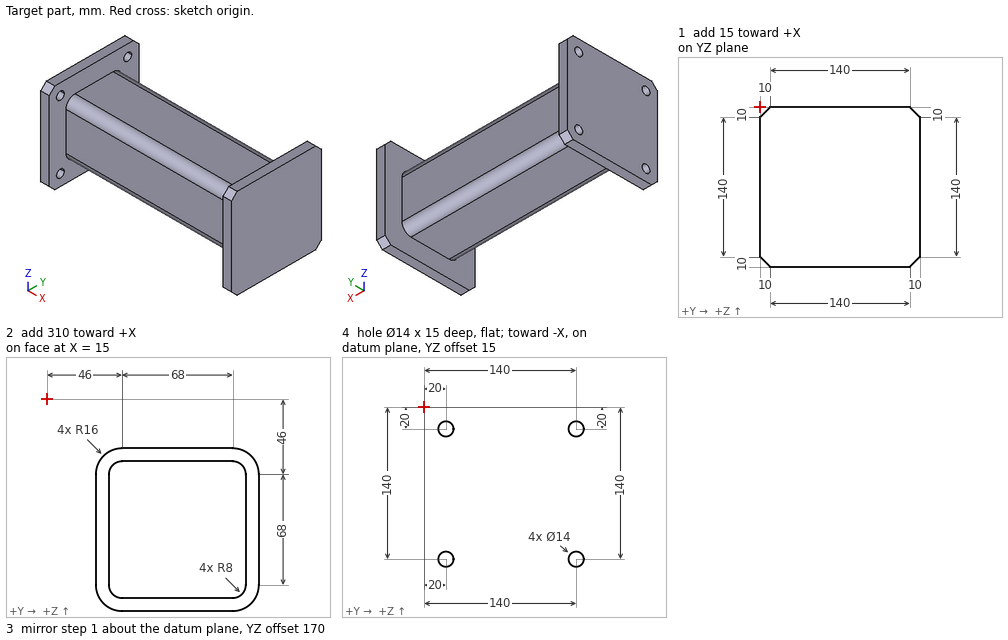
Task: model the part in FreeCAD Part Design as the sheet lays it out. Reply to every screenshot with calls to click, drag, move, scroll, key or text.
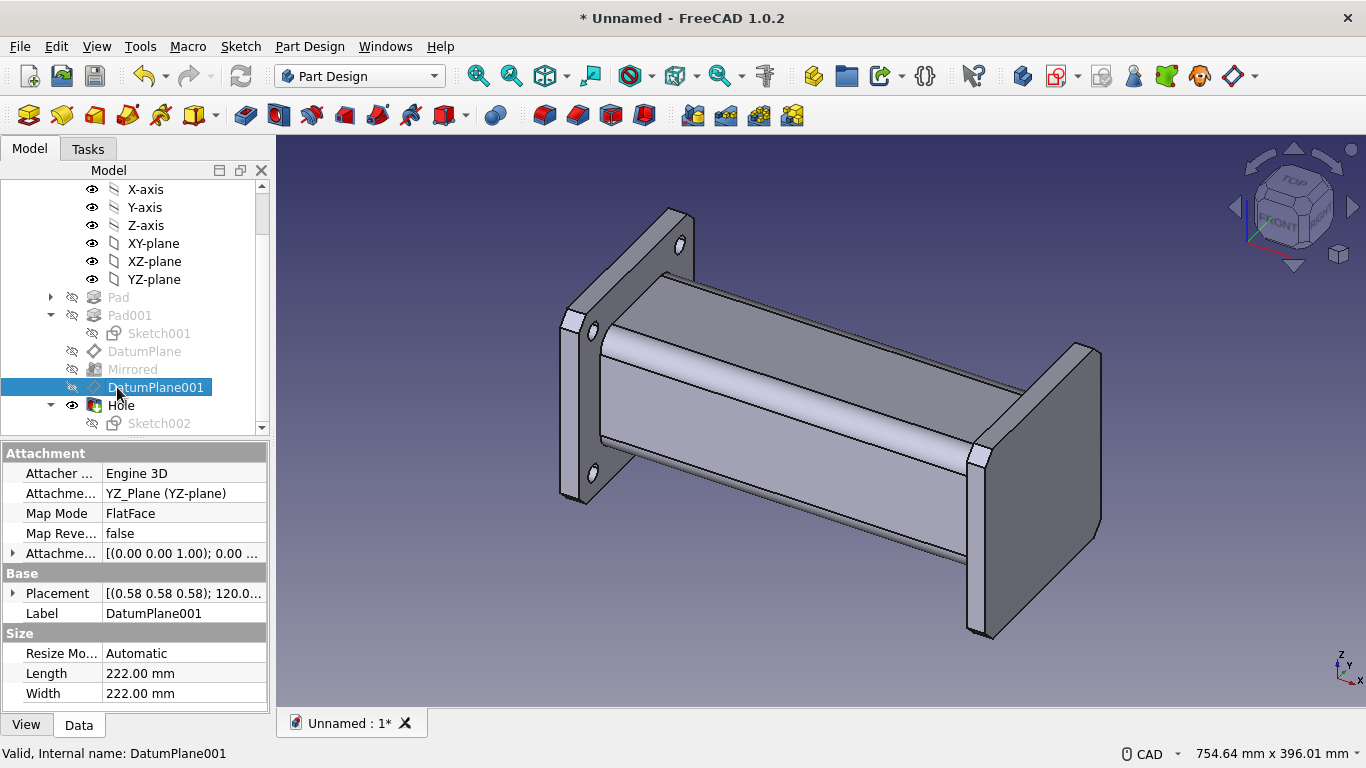
key(0)